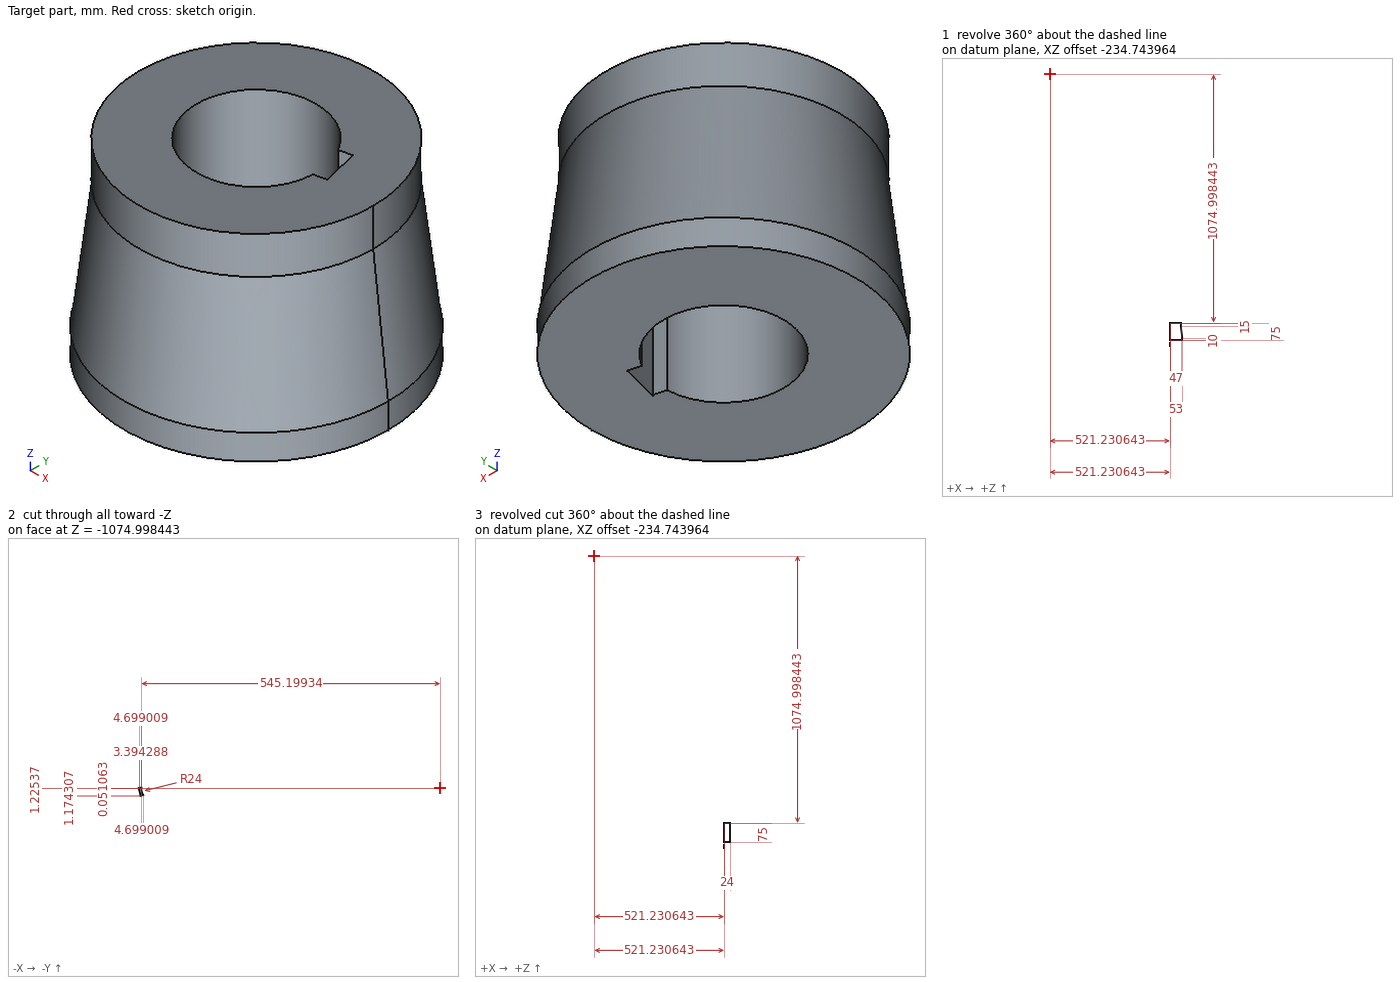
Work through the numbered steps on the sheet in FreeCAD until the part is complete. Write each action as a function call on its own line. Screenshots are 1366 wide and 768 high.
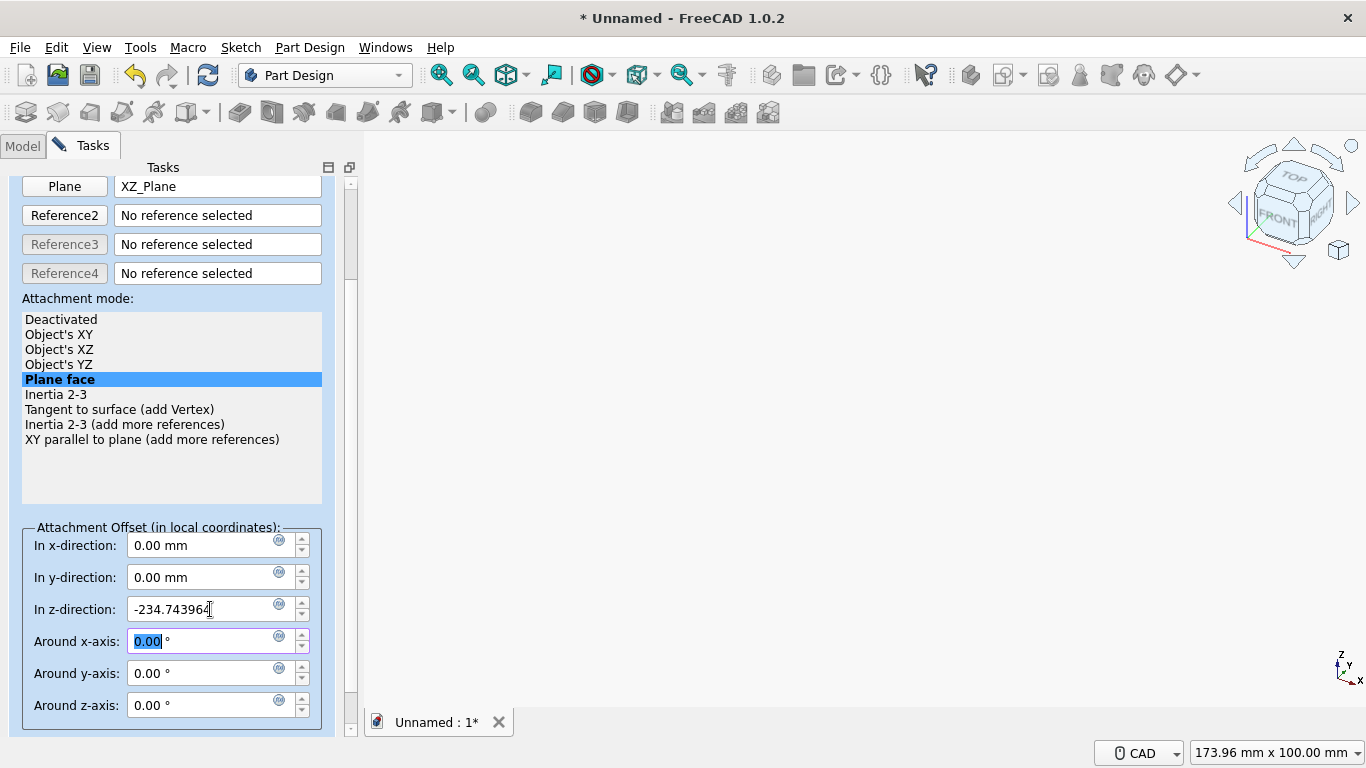
scroll(351, 456, up, 3)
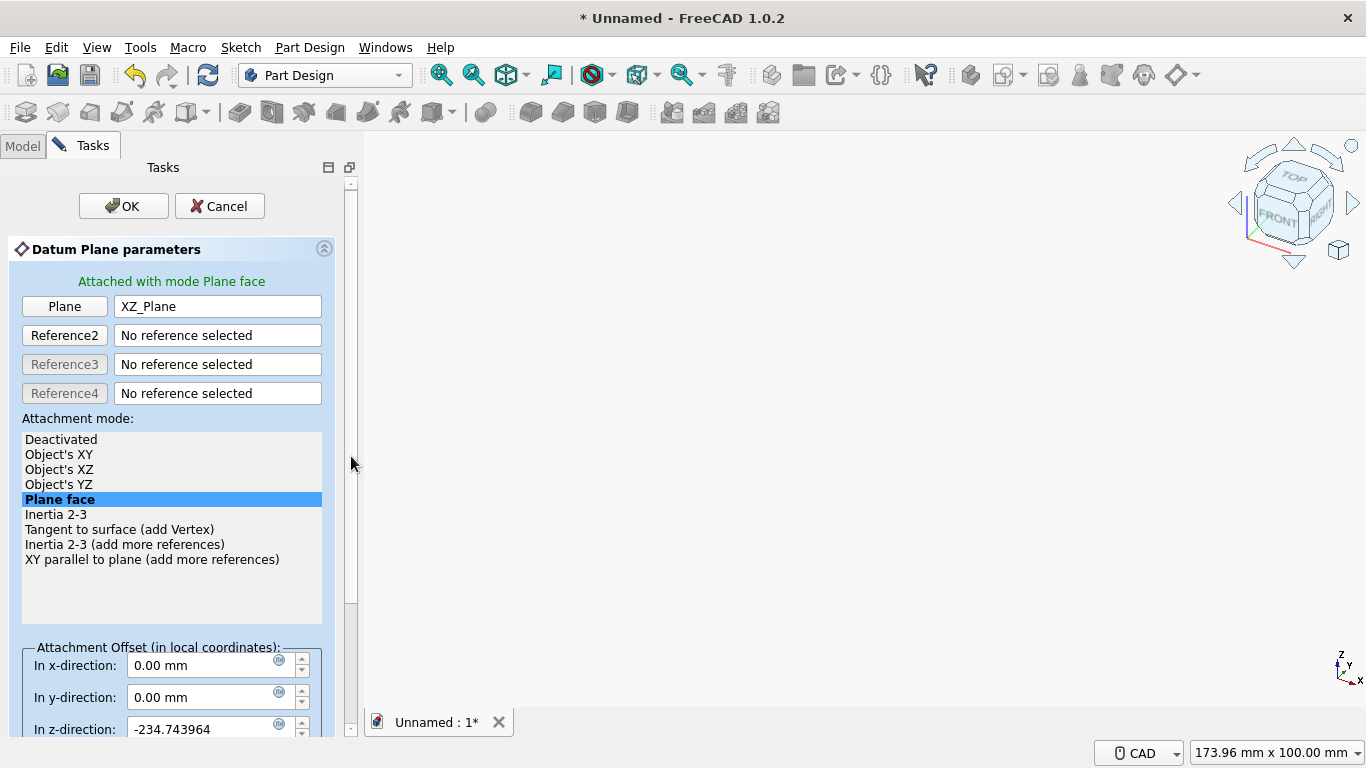
click(124, 206)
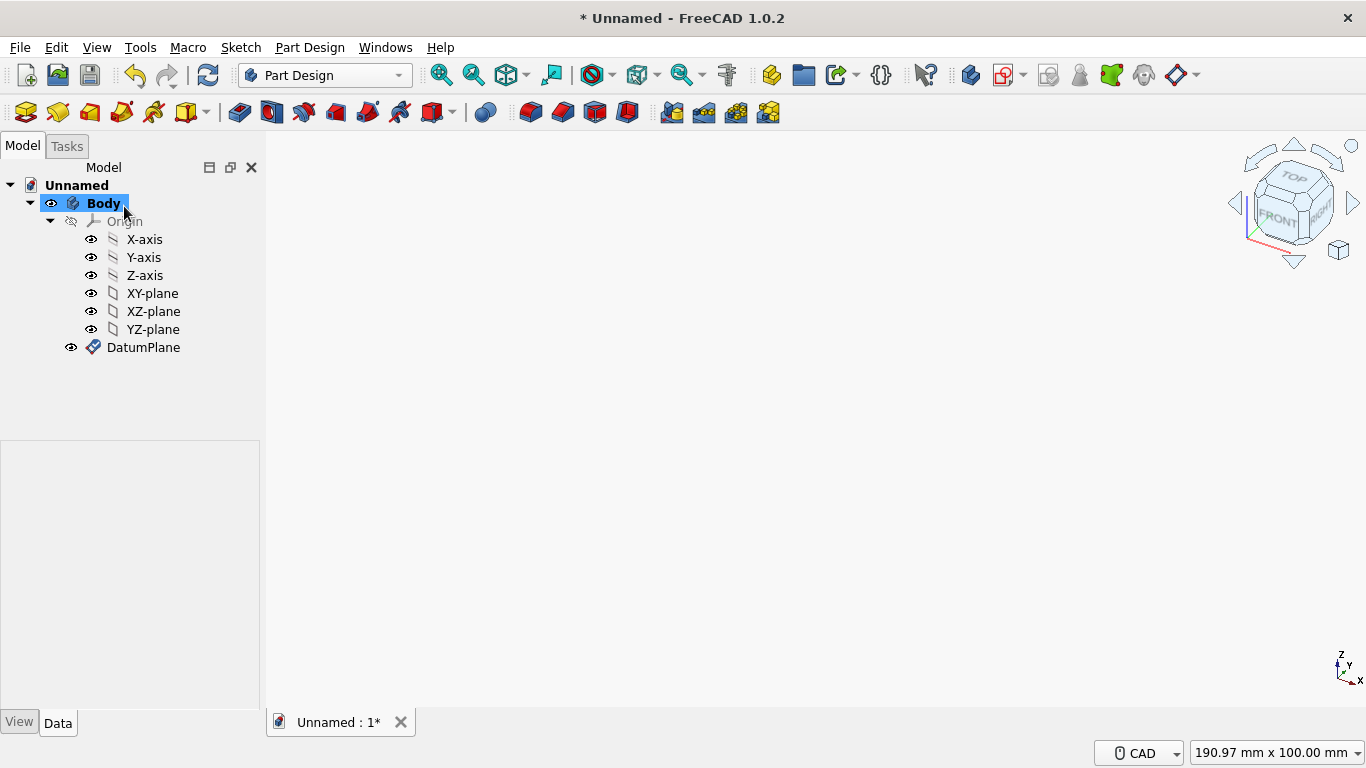
click(116, 347)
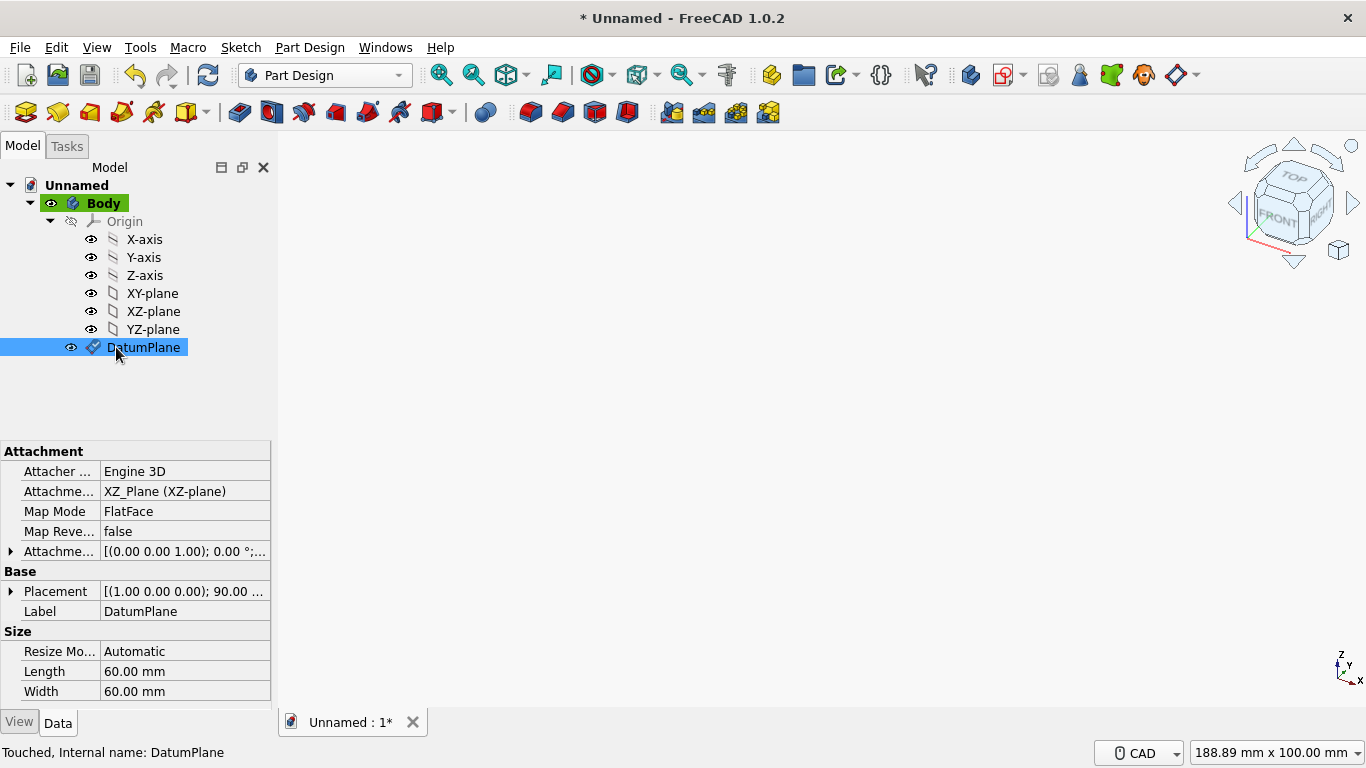
click(1004, 76)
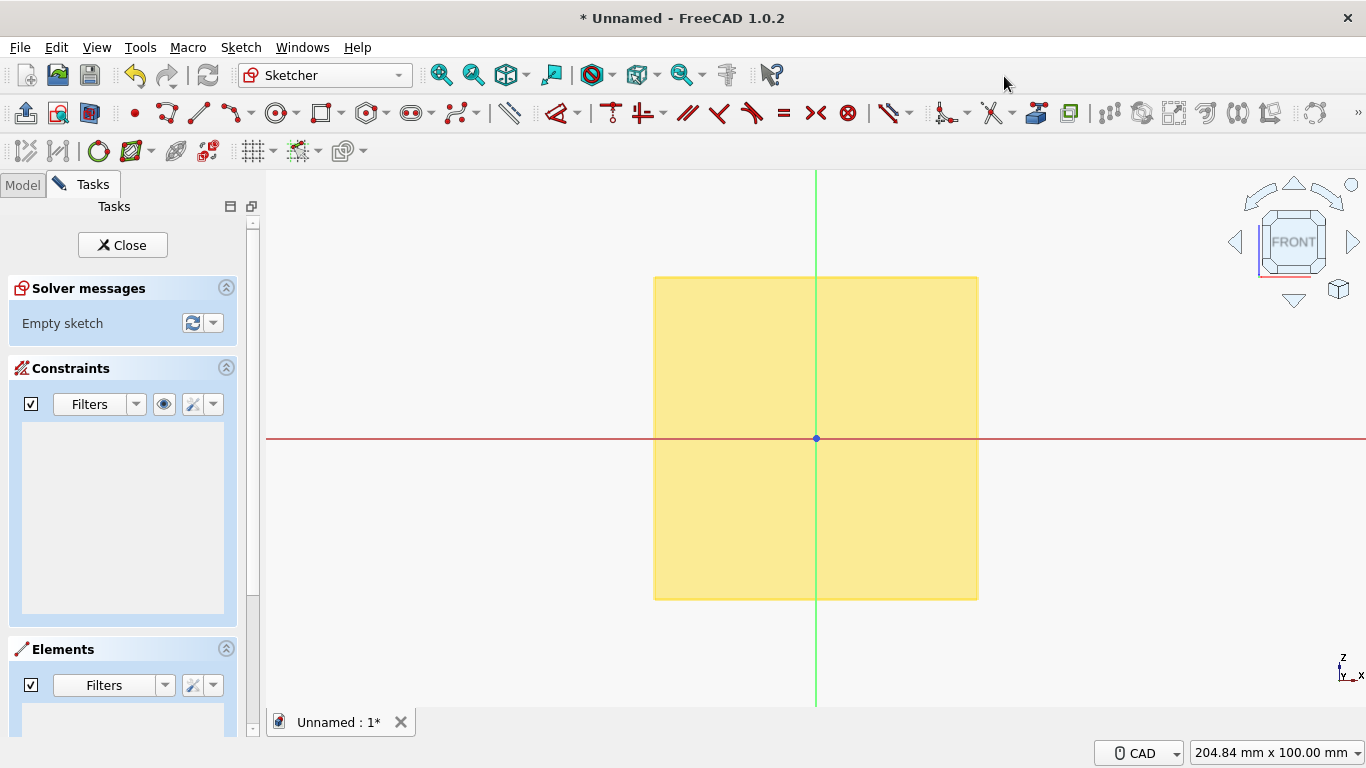
scroll(748, 438, down, 5)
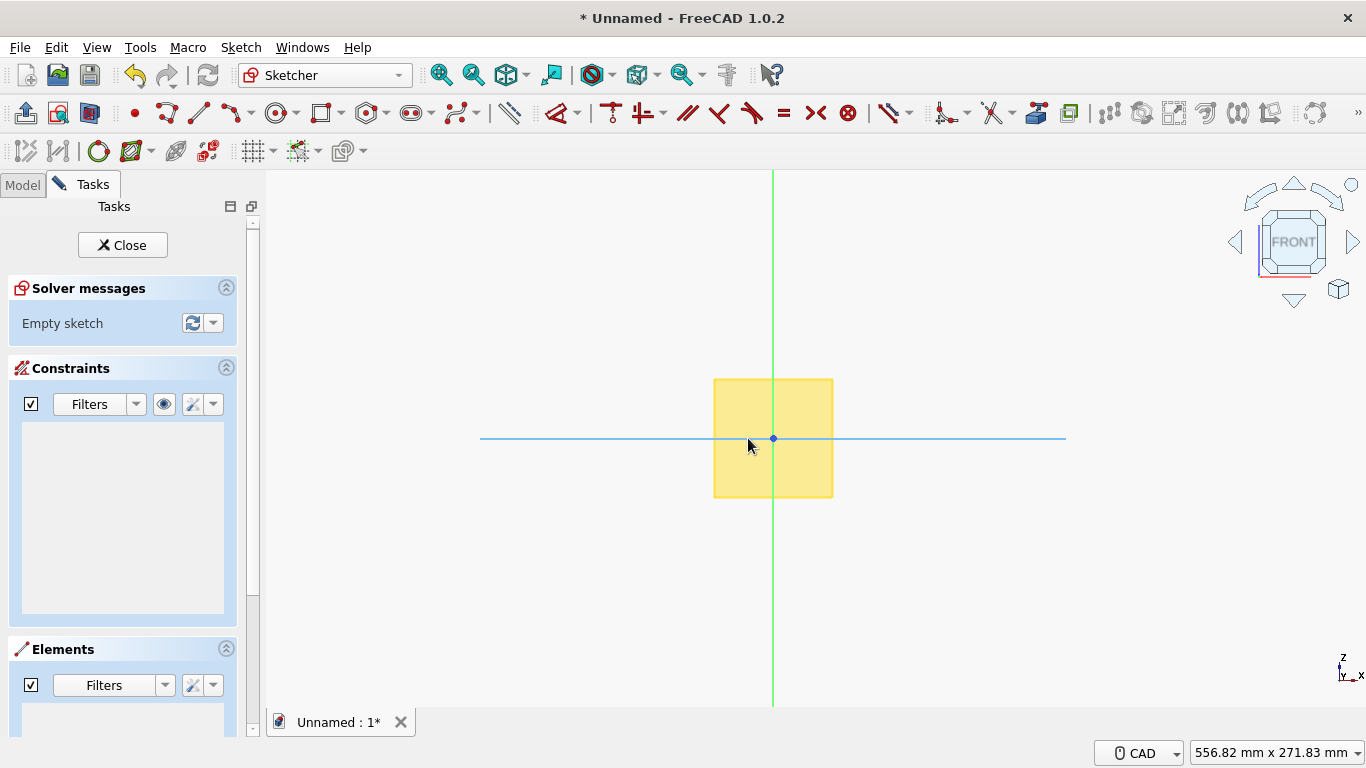
scroll(748, 438, down, 5)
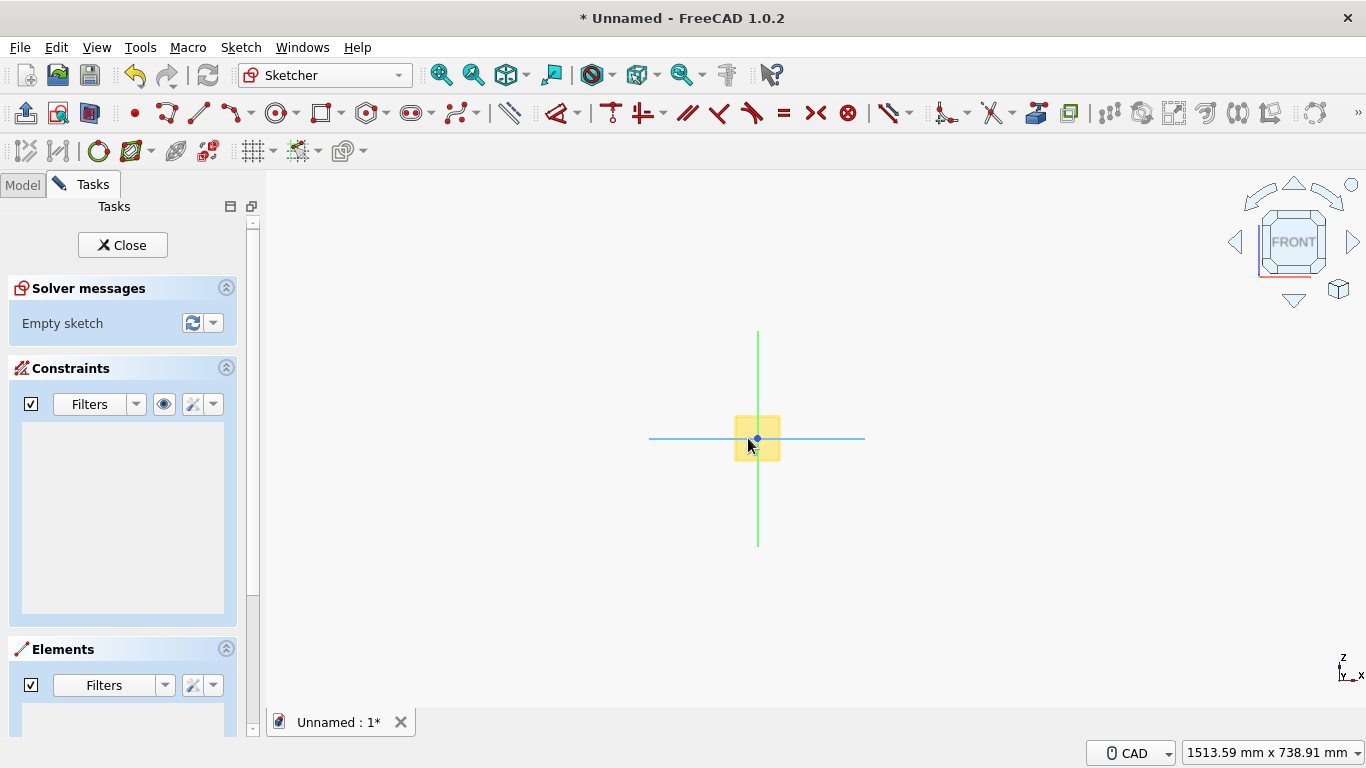
scroll(748, 438, down, 5)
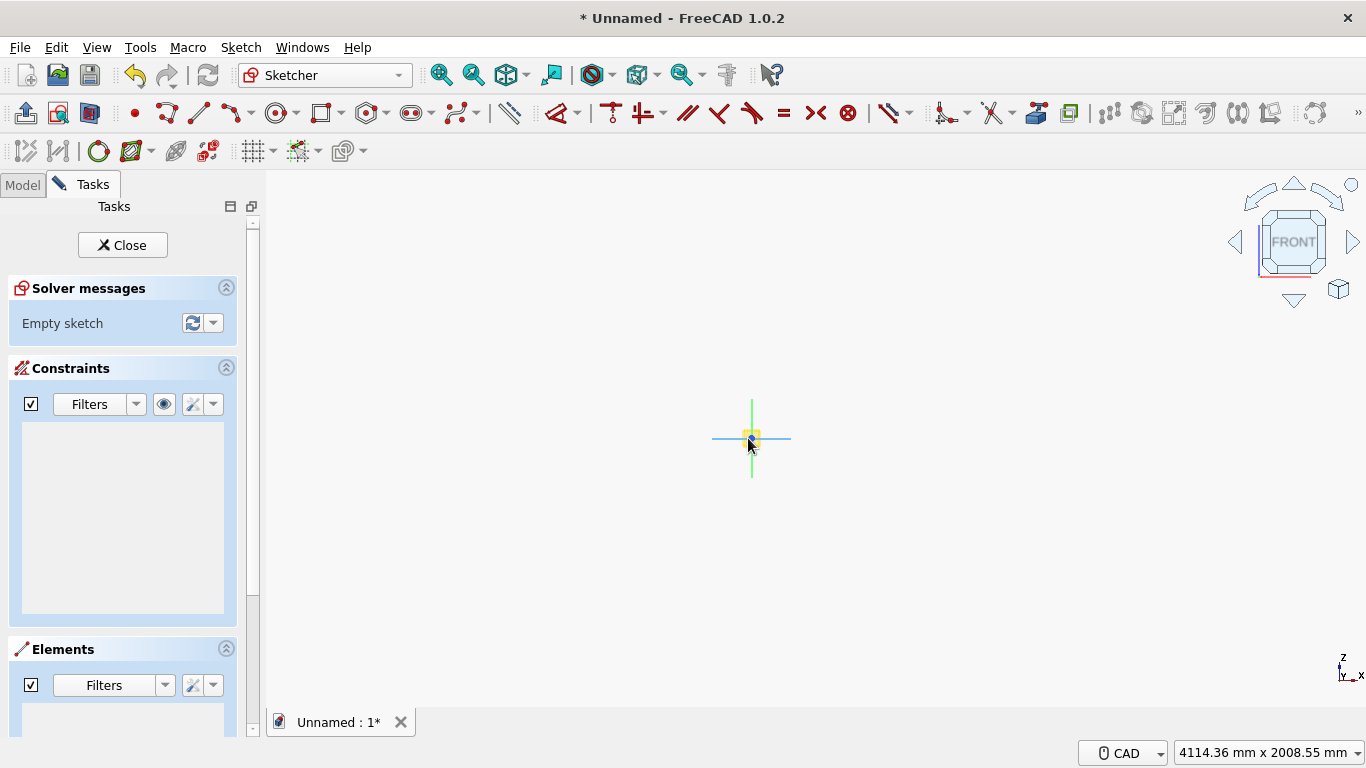
scroll(748, 438, down, 5)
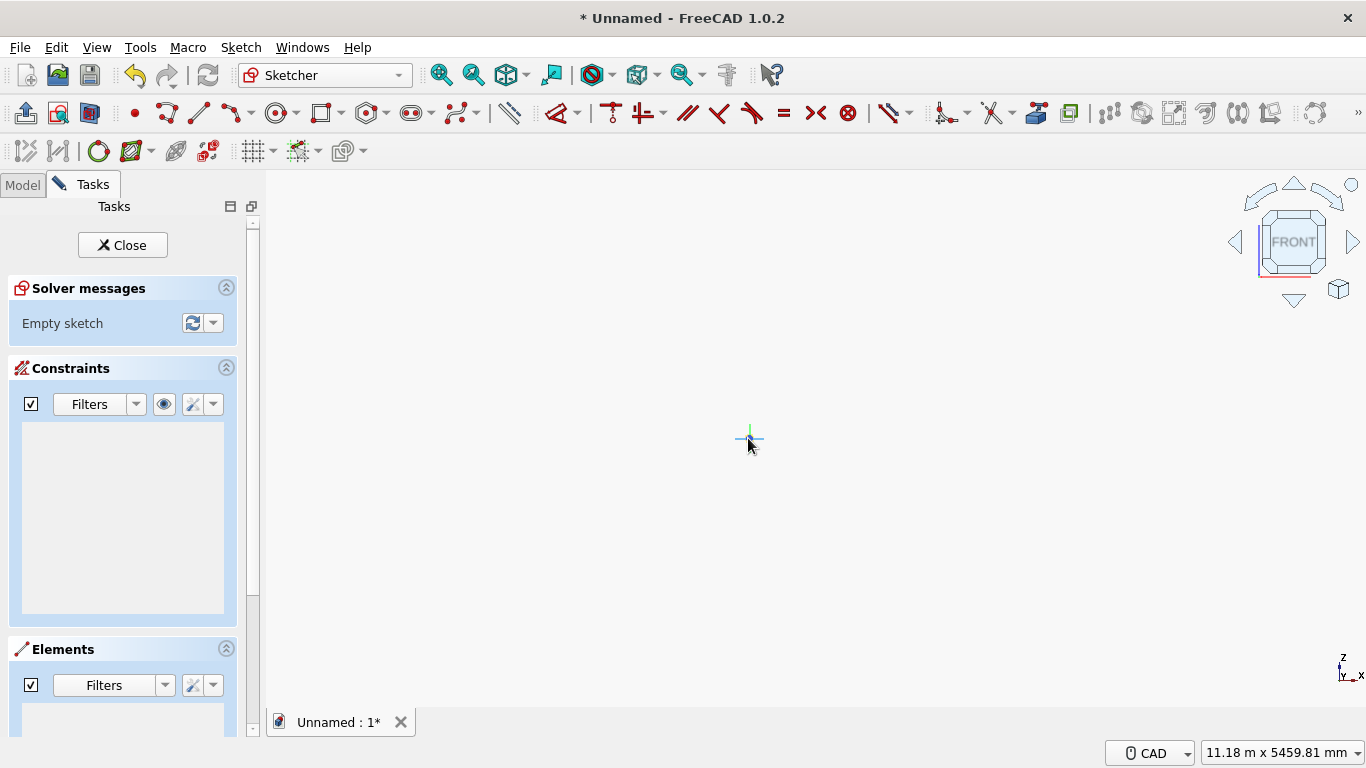
scroll(806, 555, up, 15)